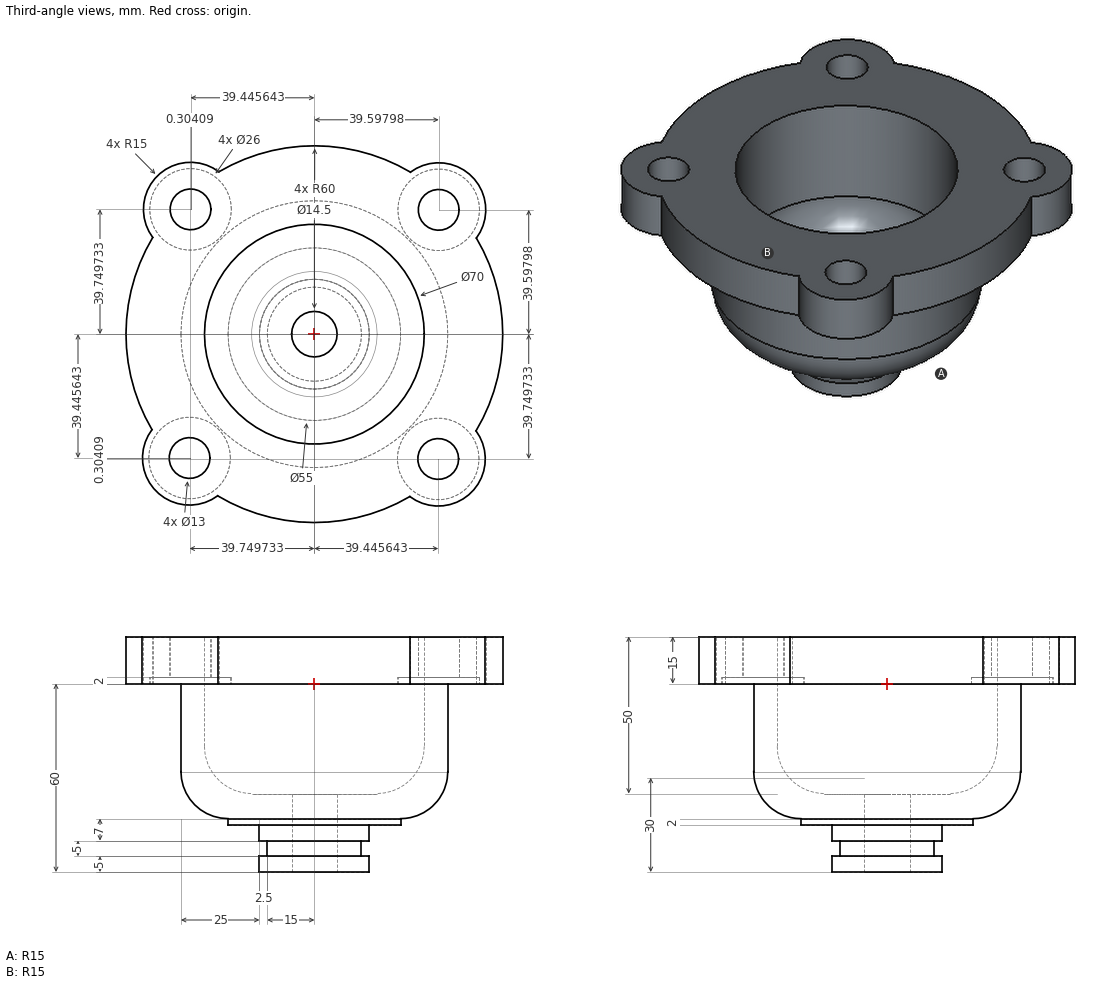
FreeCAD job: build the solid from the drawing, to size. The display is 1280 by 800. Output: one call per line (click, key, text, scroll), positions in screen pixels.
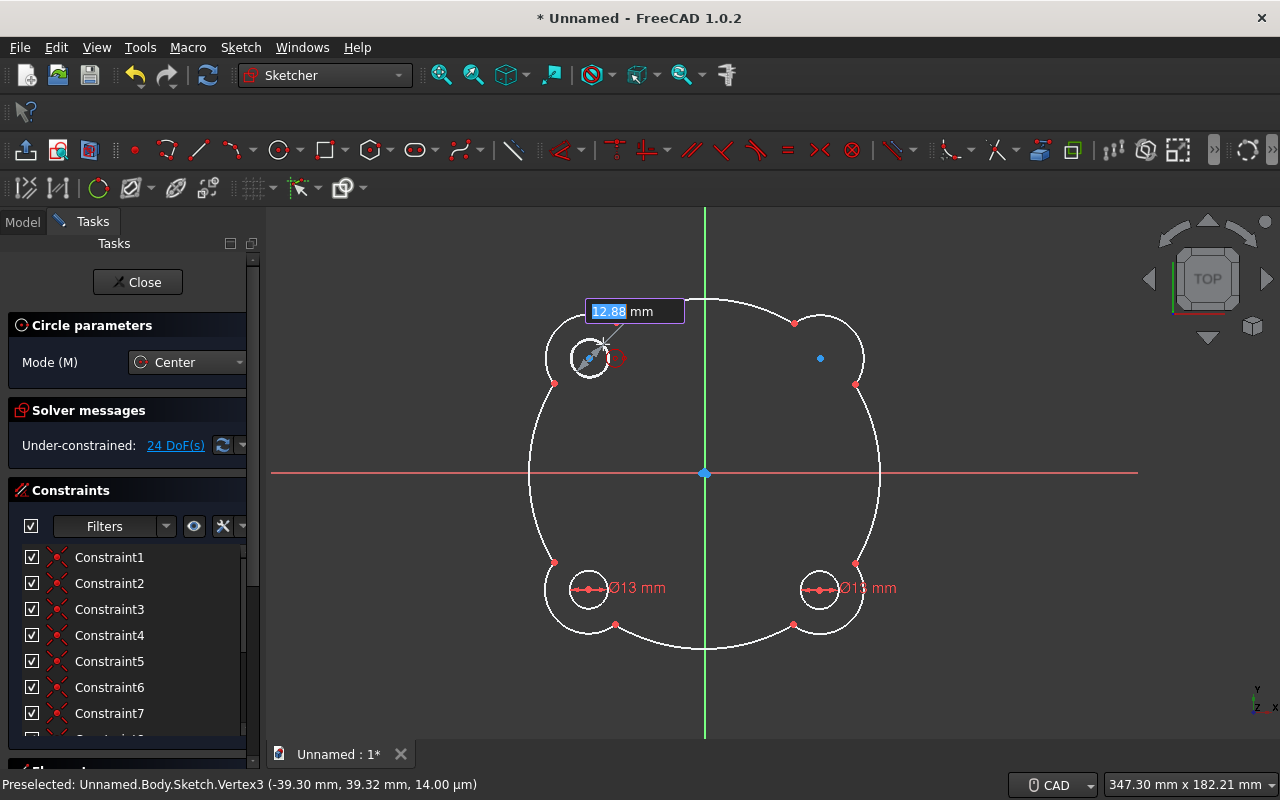
text(13)
key(Return)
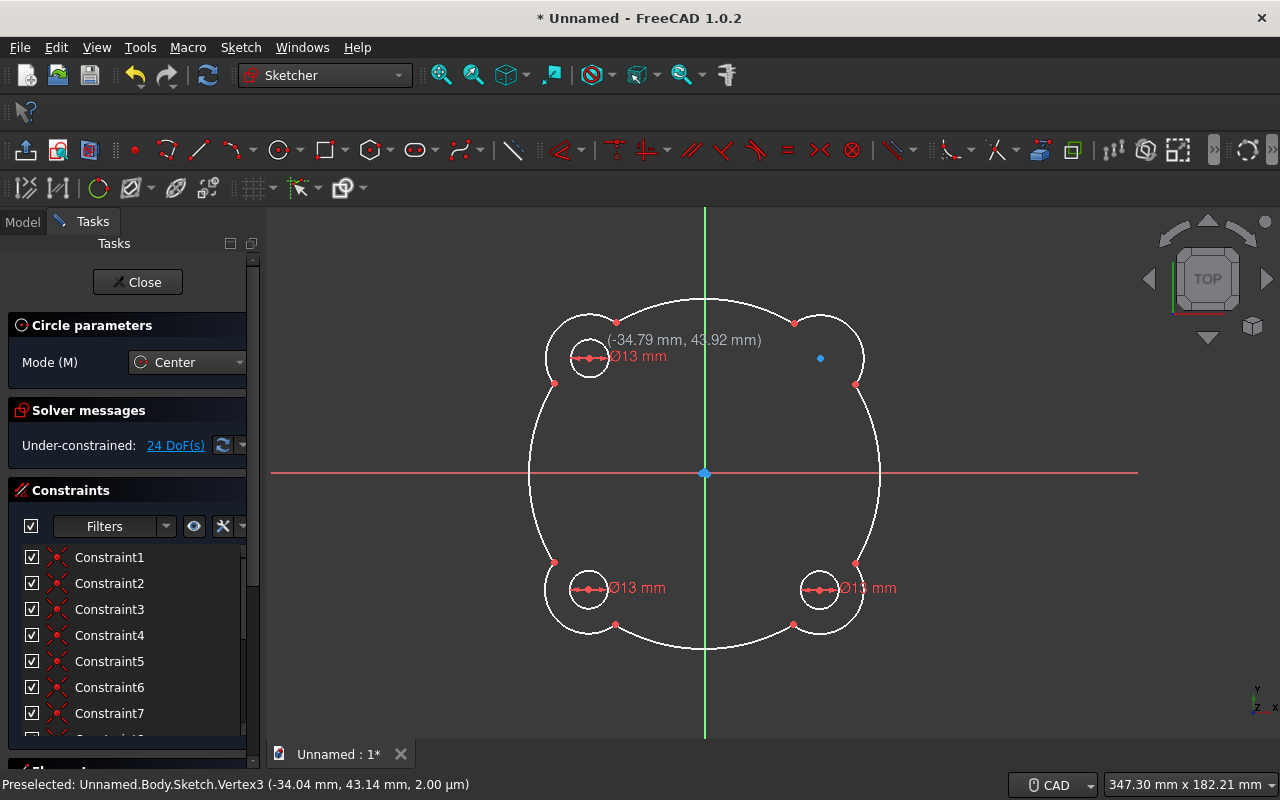
click(820, 358)
move(834, 344)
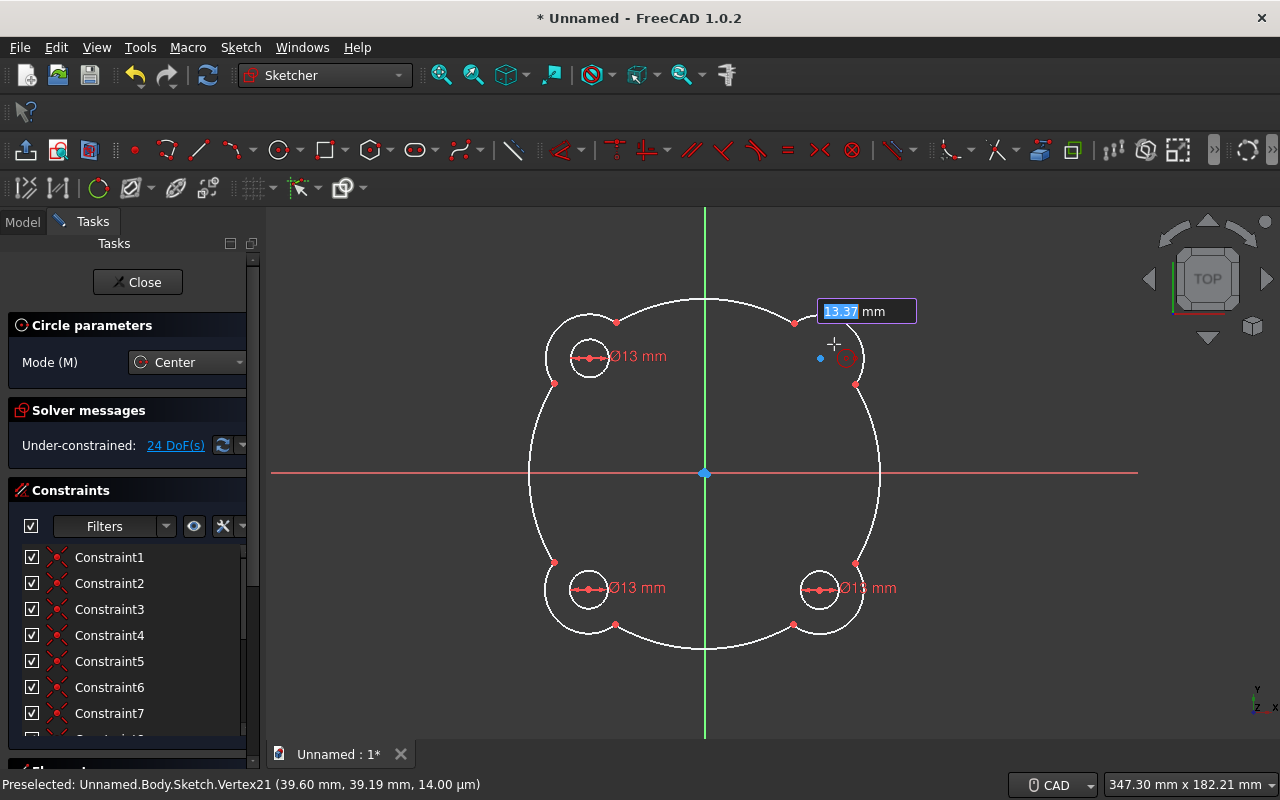
text(13)
key(Return)
key(Escape)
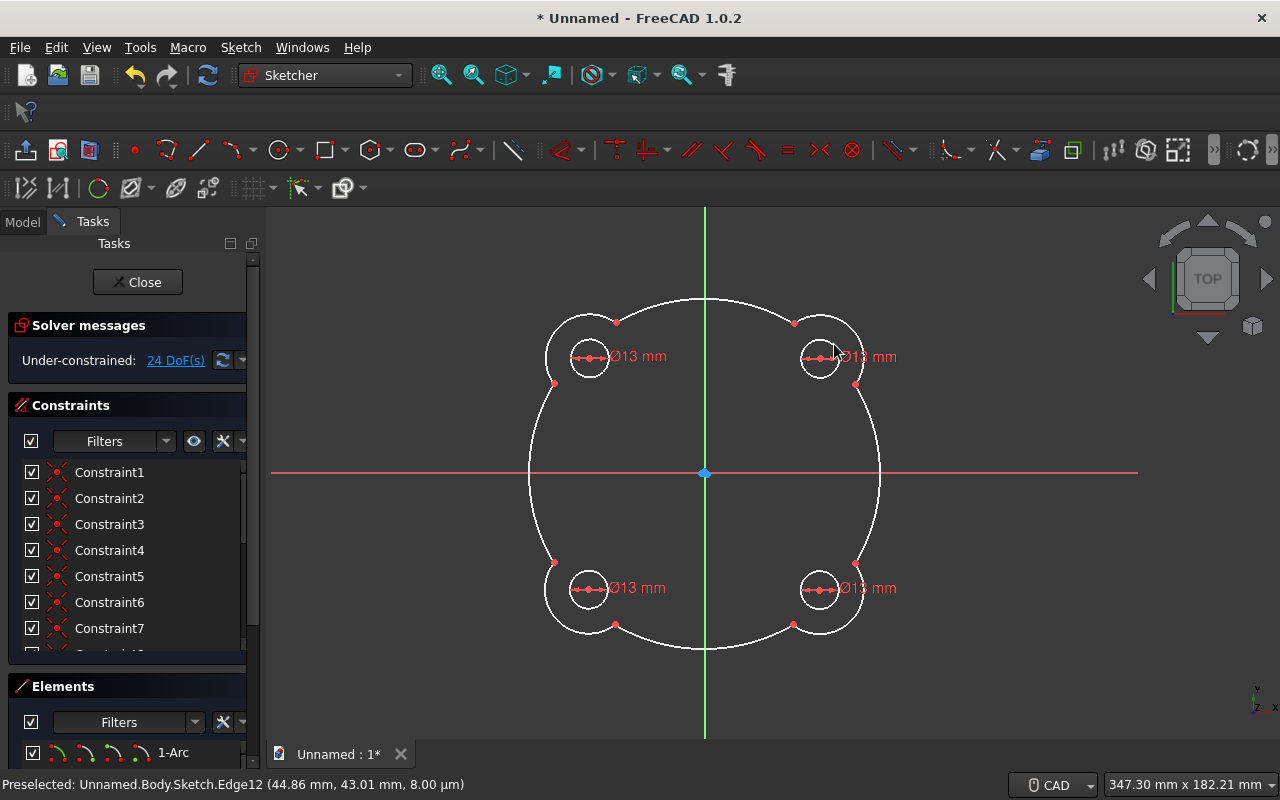
click(533, 436)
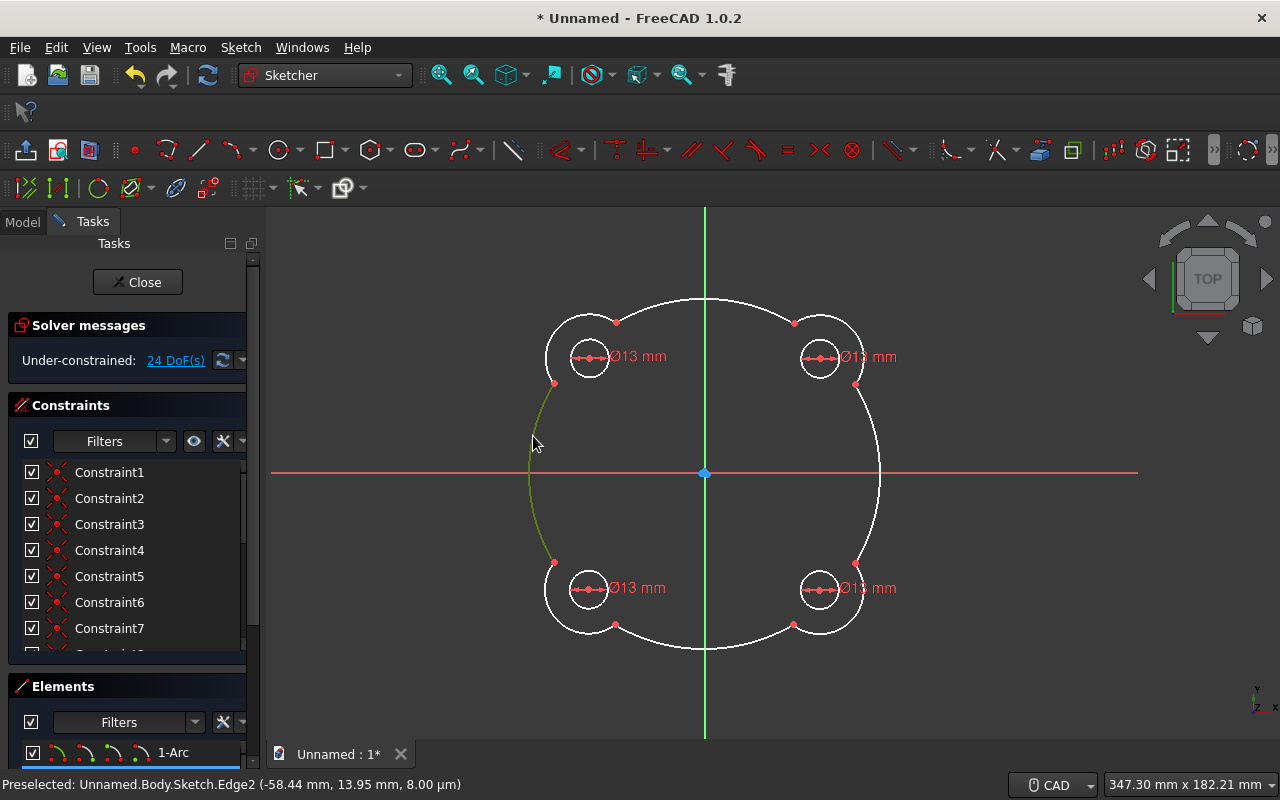
click(667, 645)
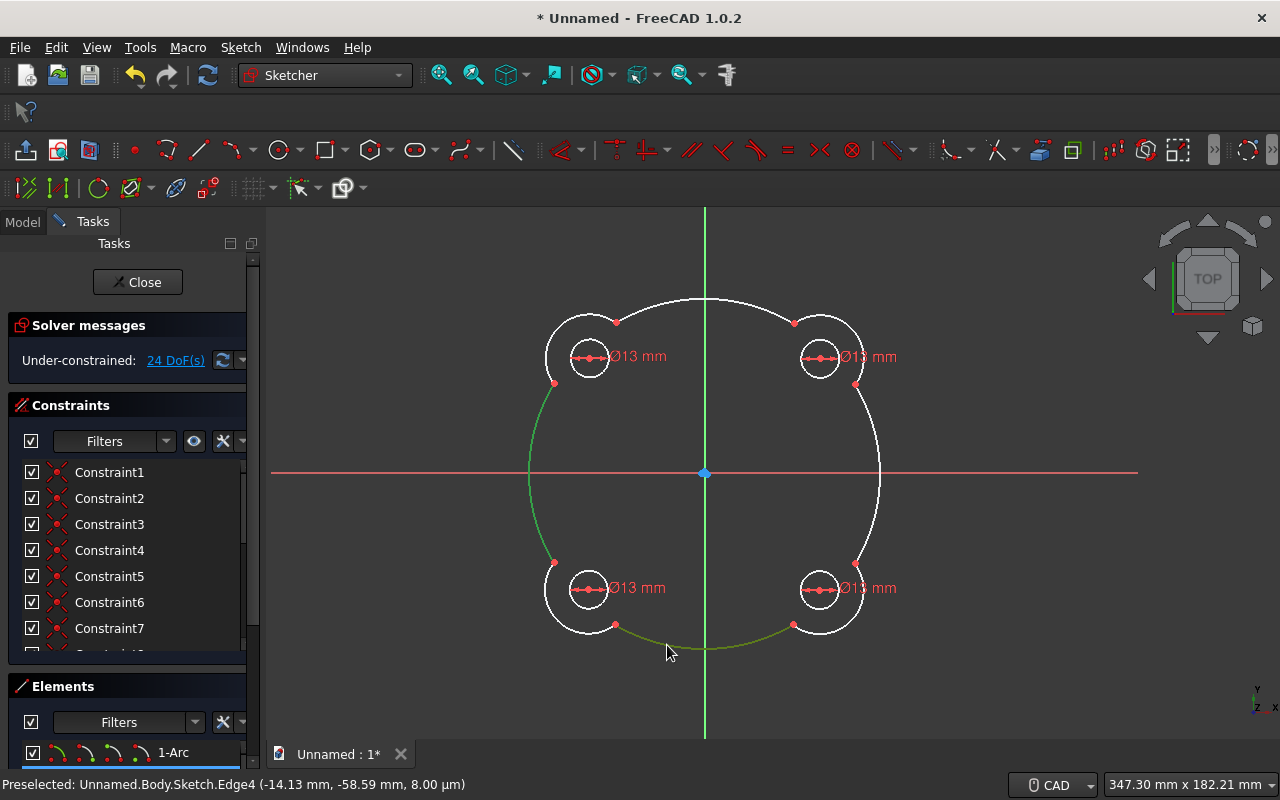
click(616, 150)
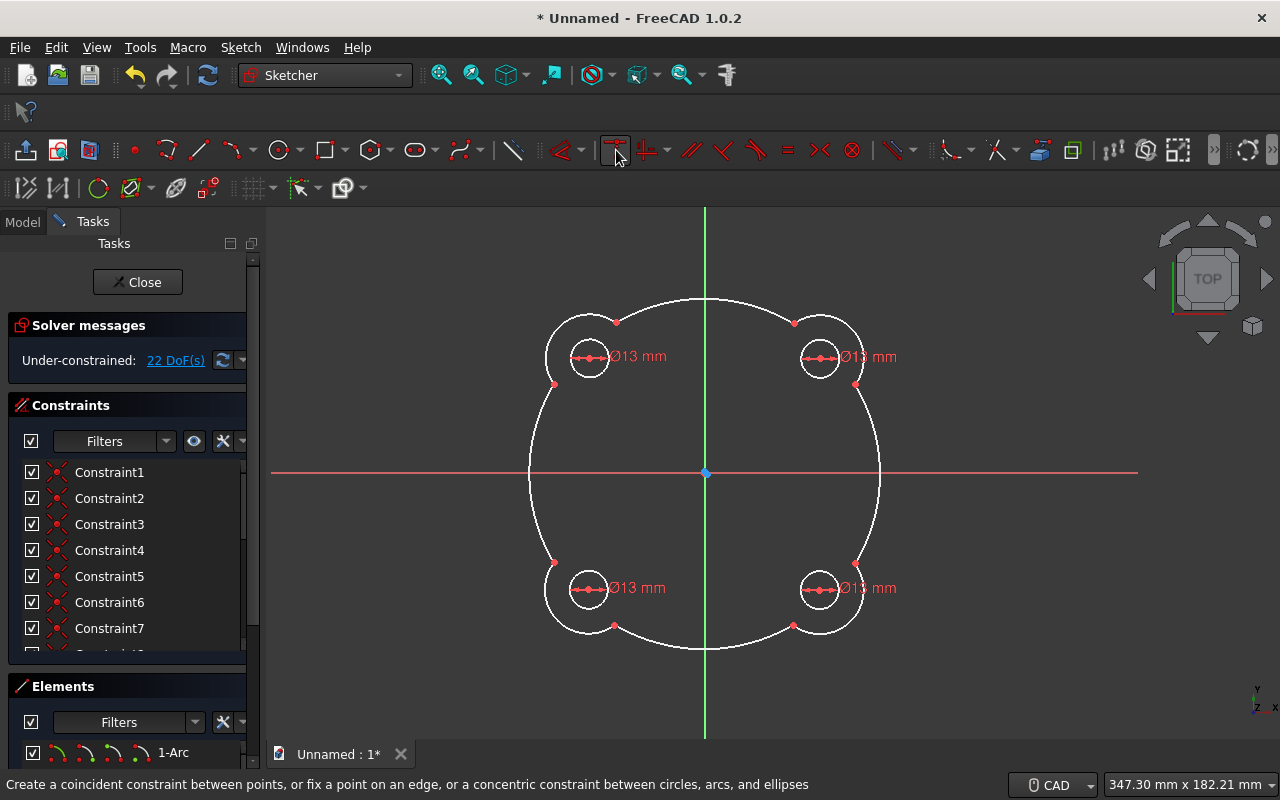
click(533, 436)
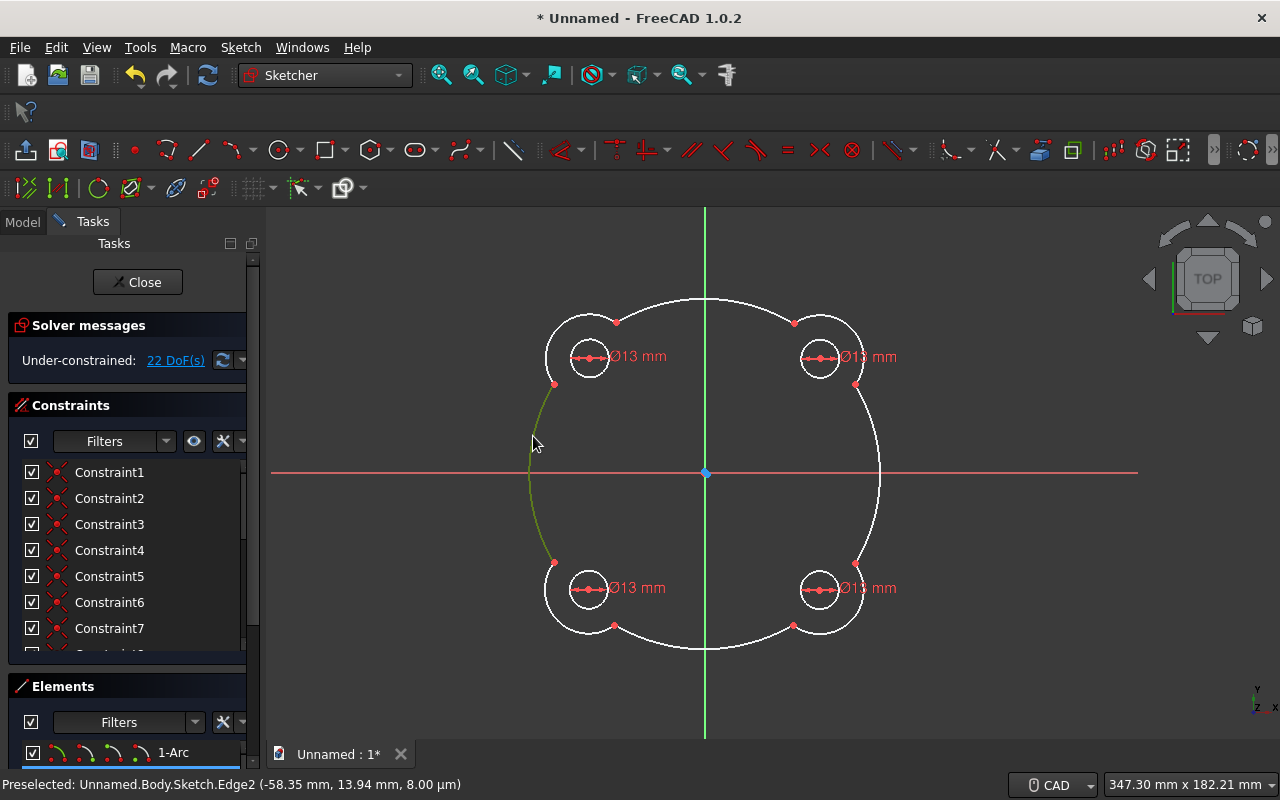
click(876, 512)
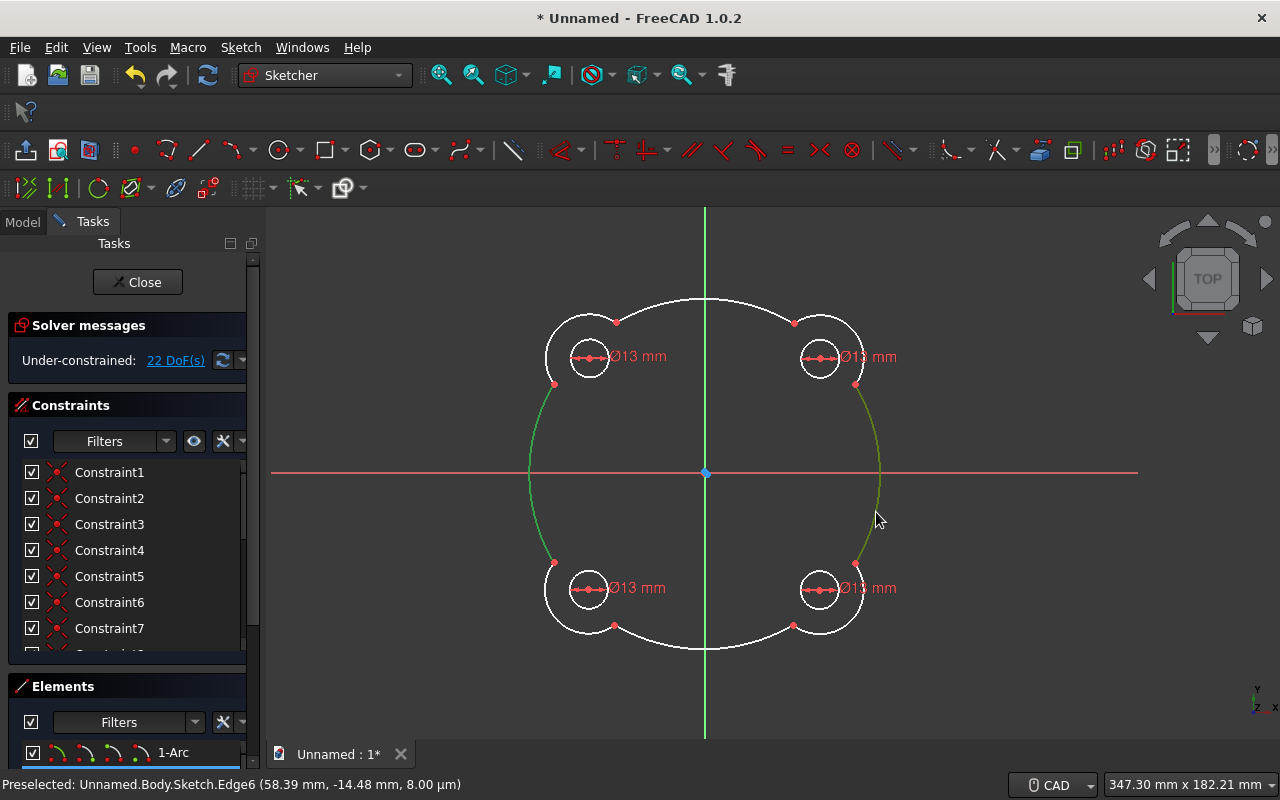
key(c)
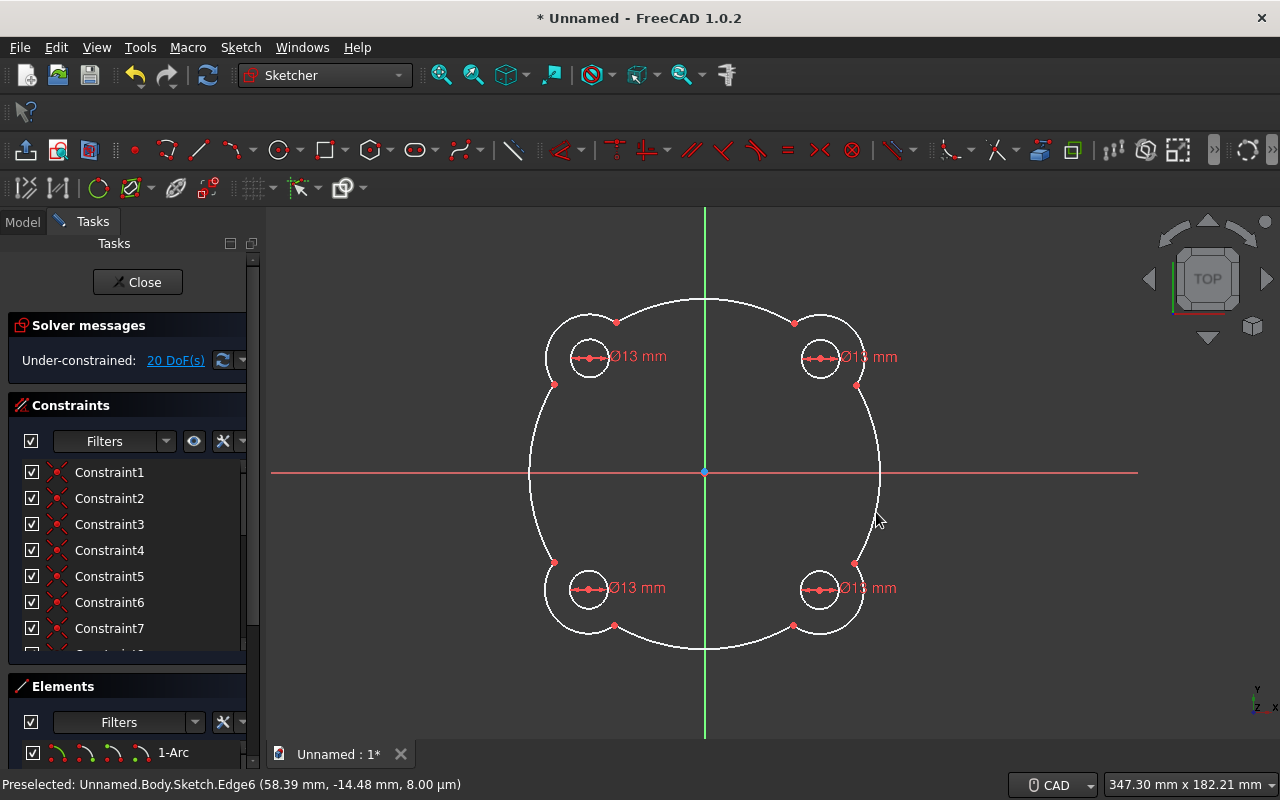
click(533, 436)